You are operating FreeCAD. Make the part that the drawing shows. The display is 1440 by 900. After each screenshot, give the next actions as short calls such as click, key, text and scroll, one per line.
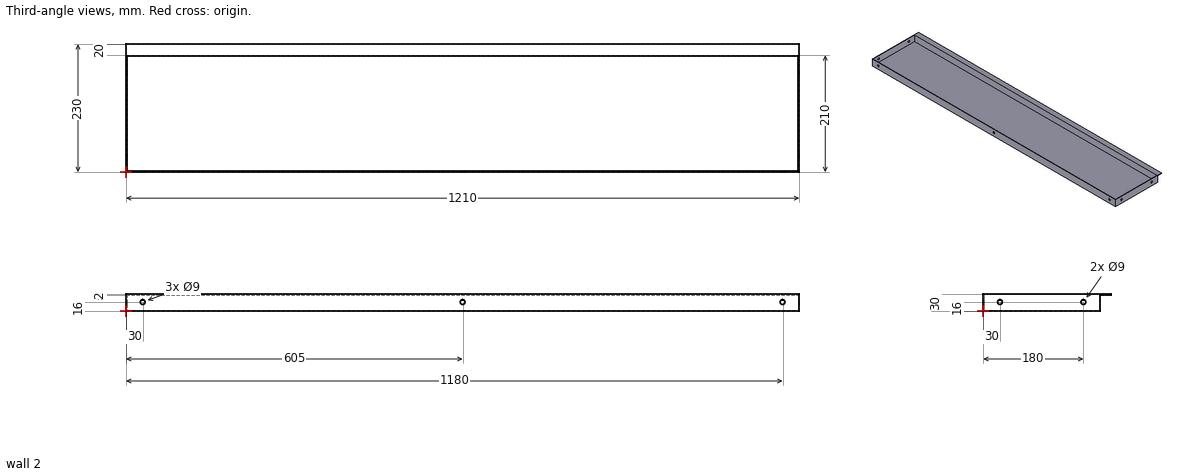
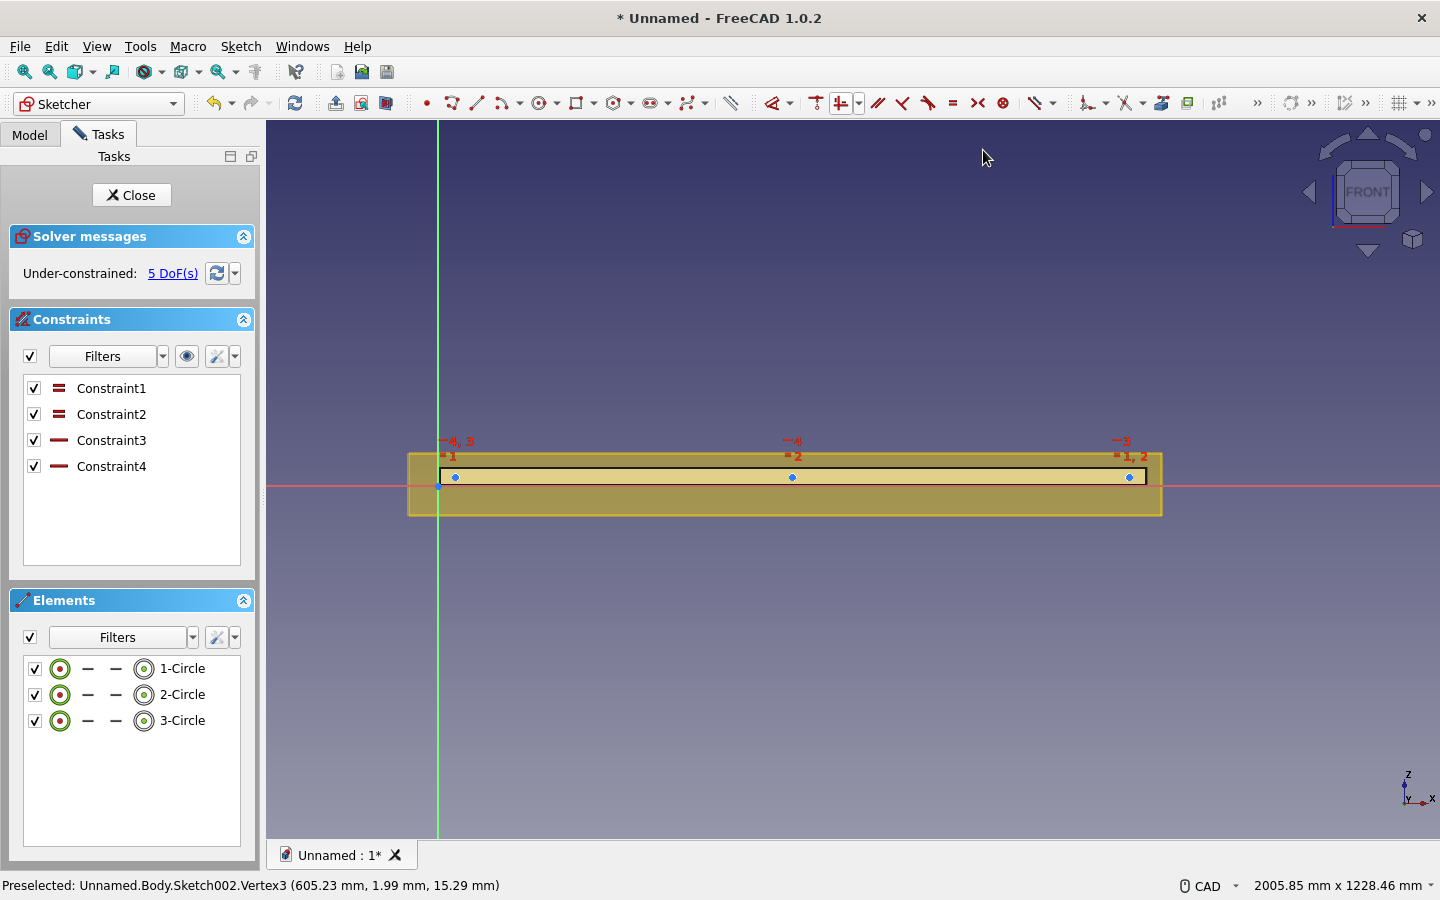
click(772, 104)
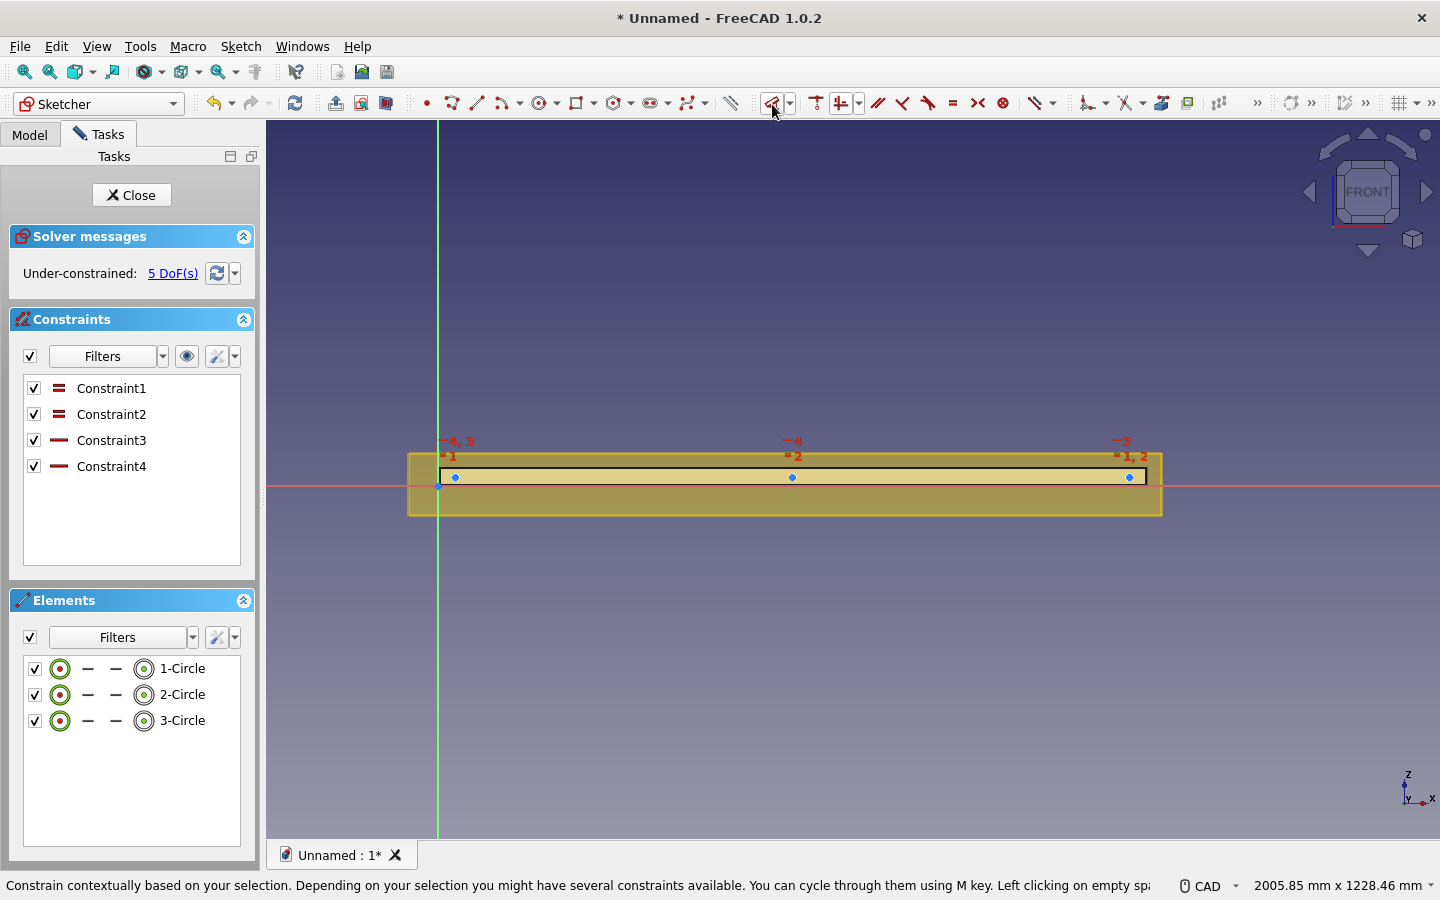
scroll(454, 475, up, 11)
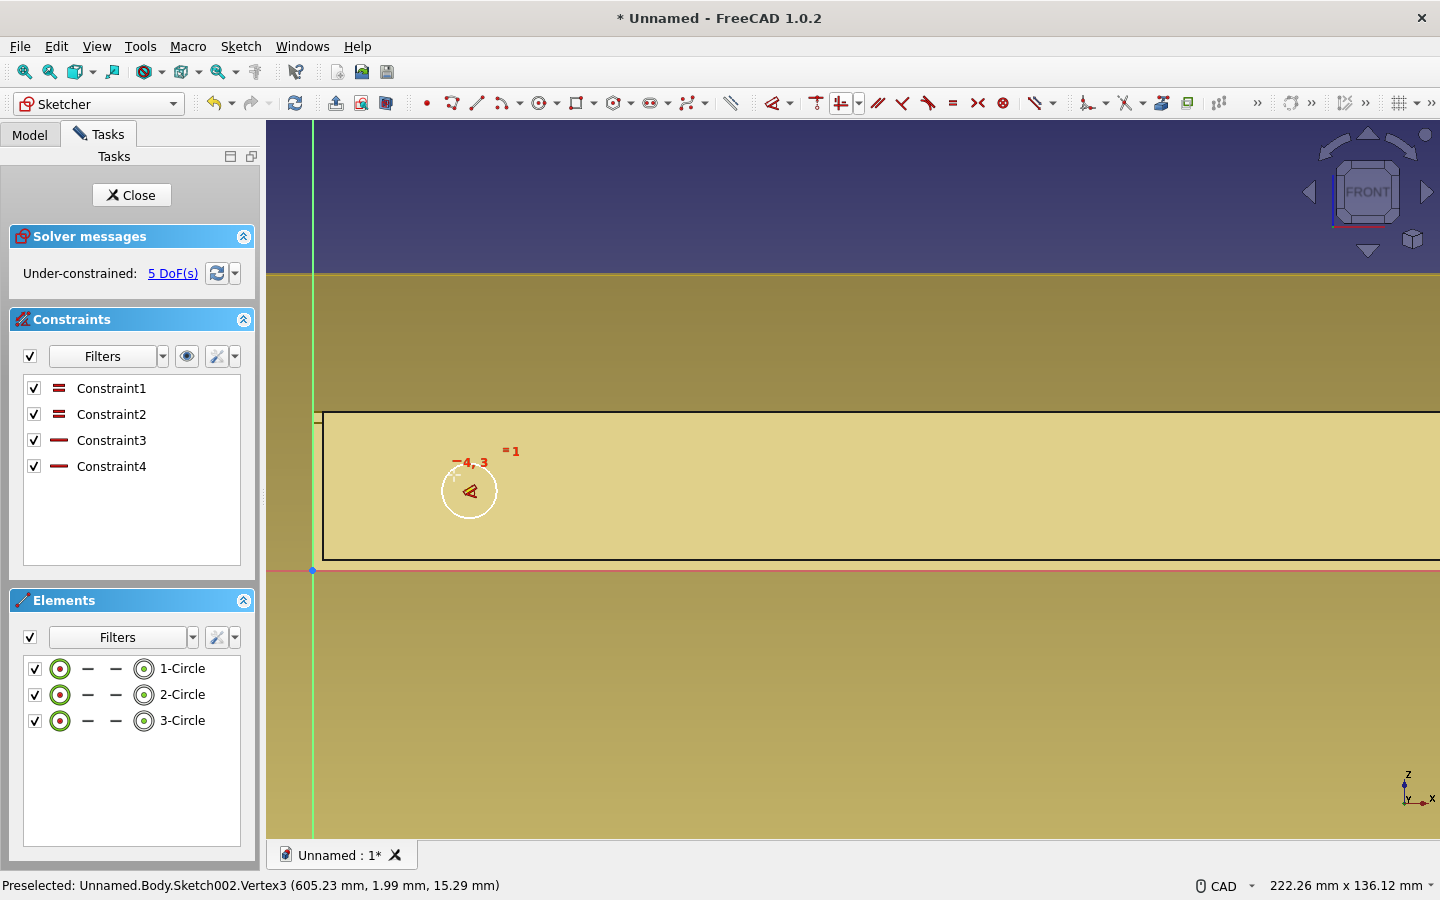
click(450, 472)
click(427, 450)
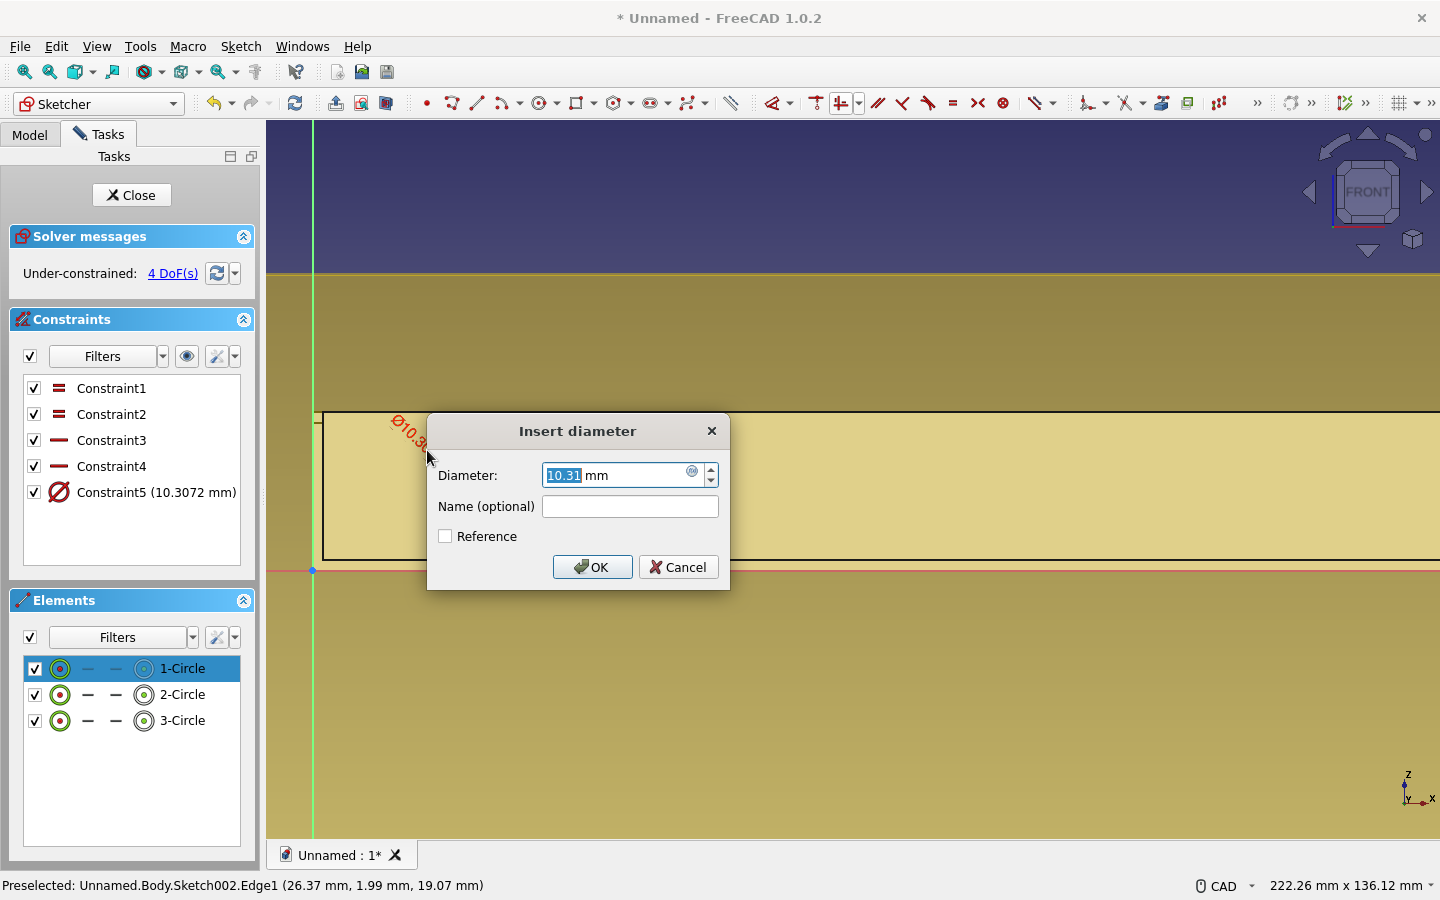
text(9)
key(Return)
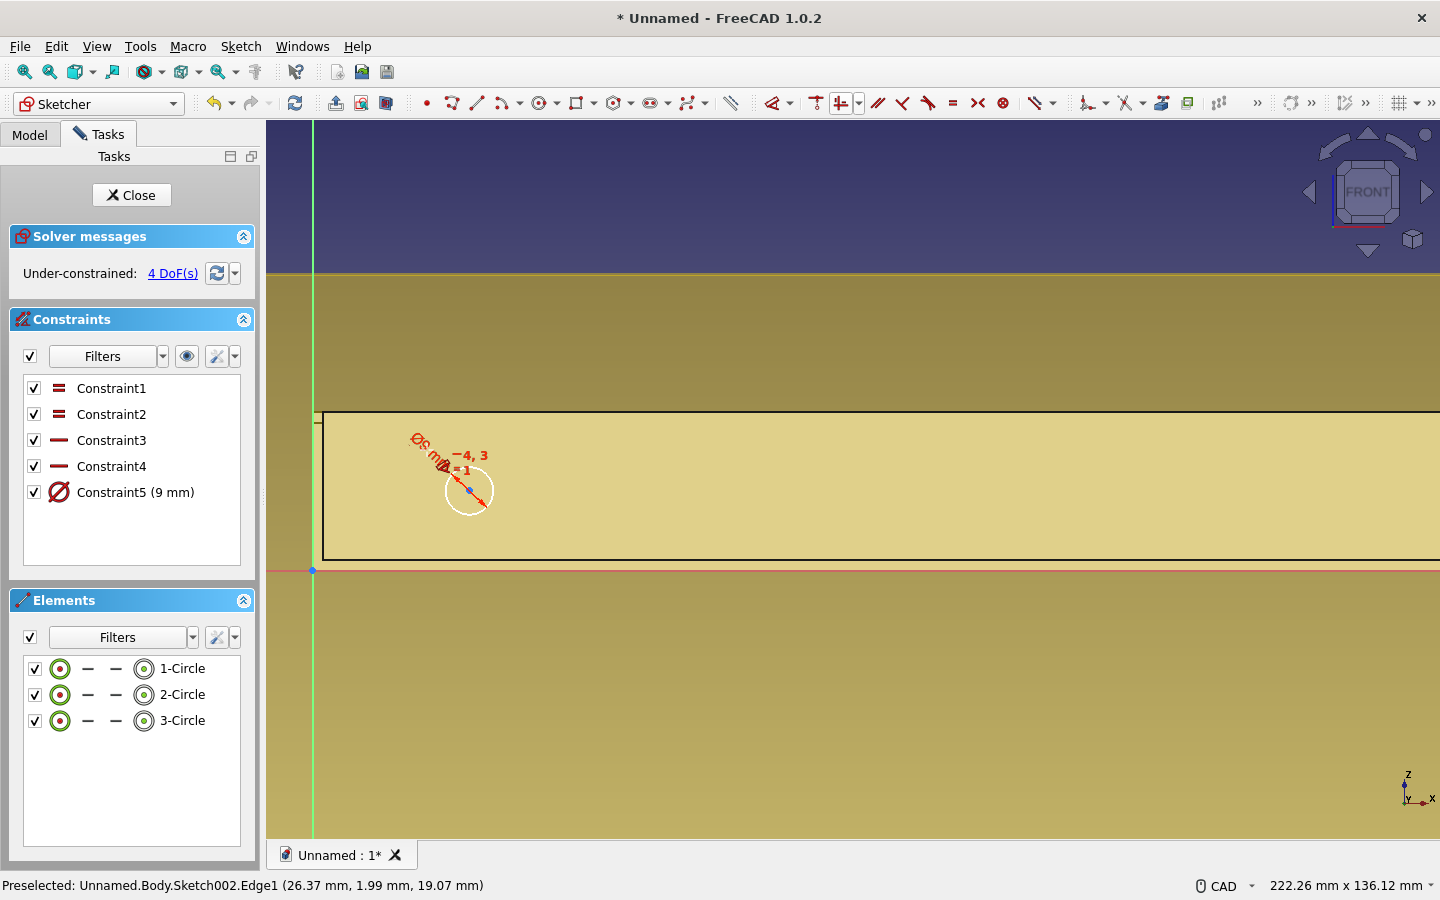
scroll(453, 475, down, 11)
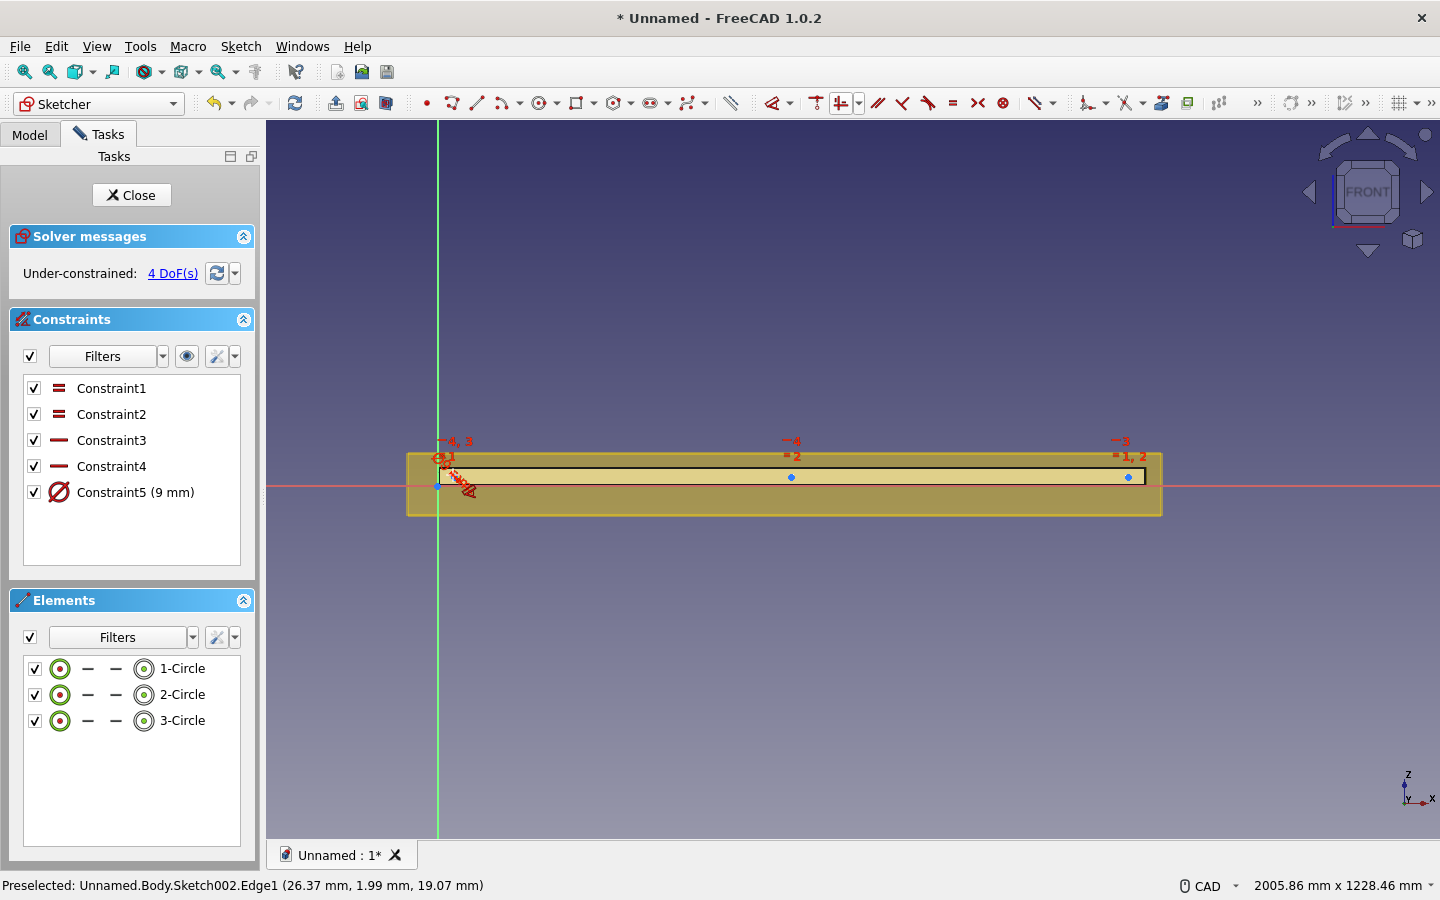
scroll(455, 477, up, 5)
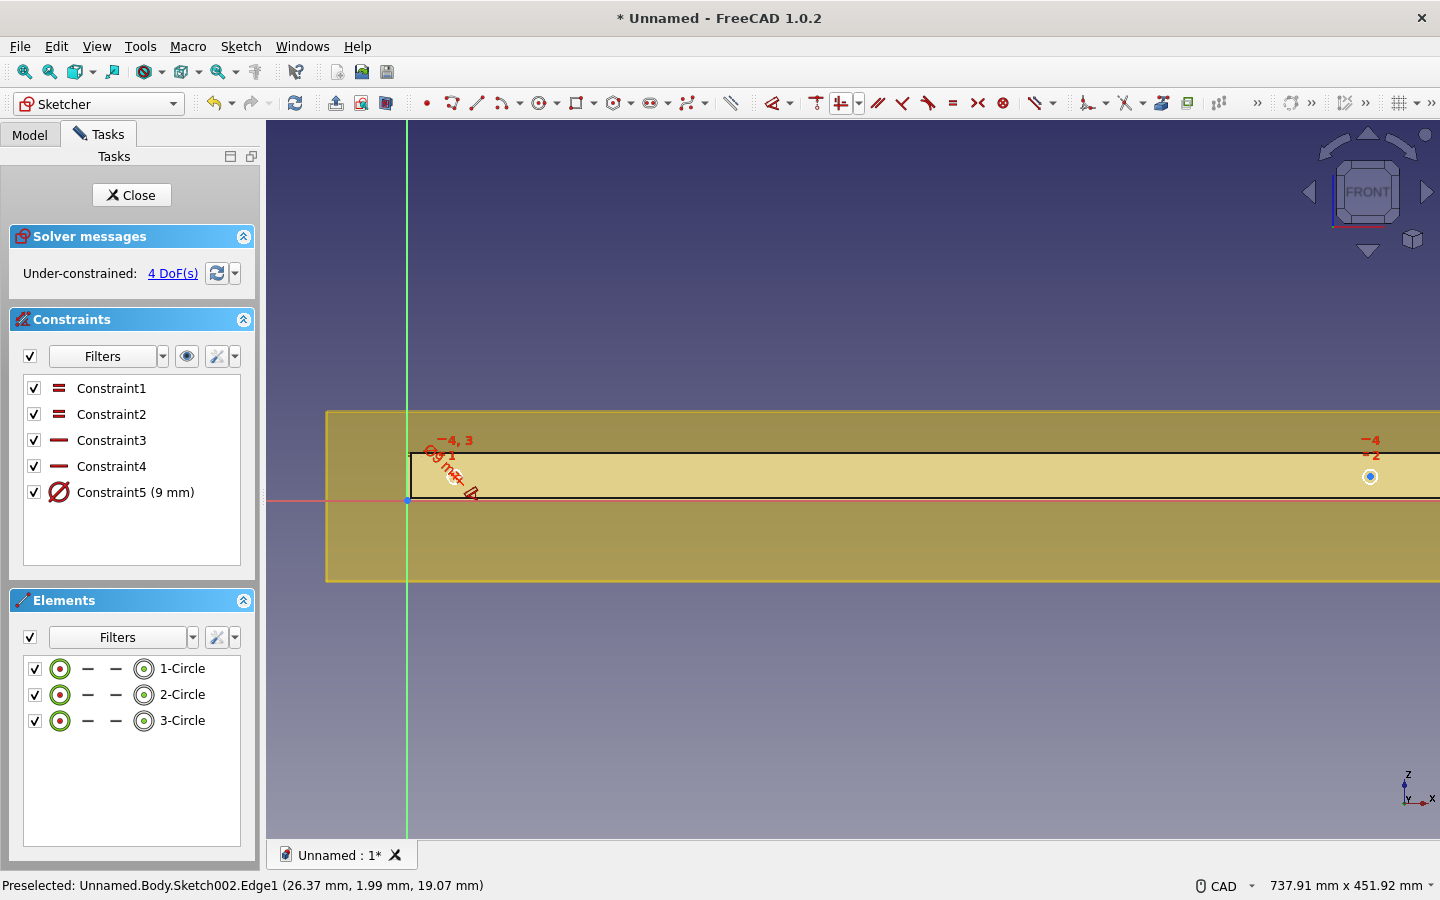
click(455, 477)
click(431, 535)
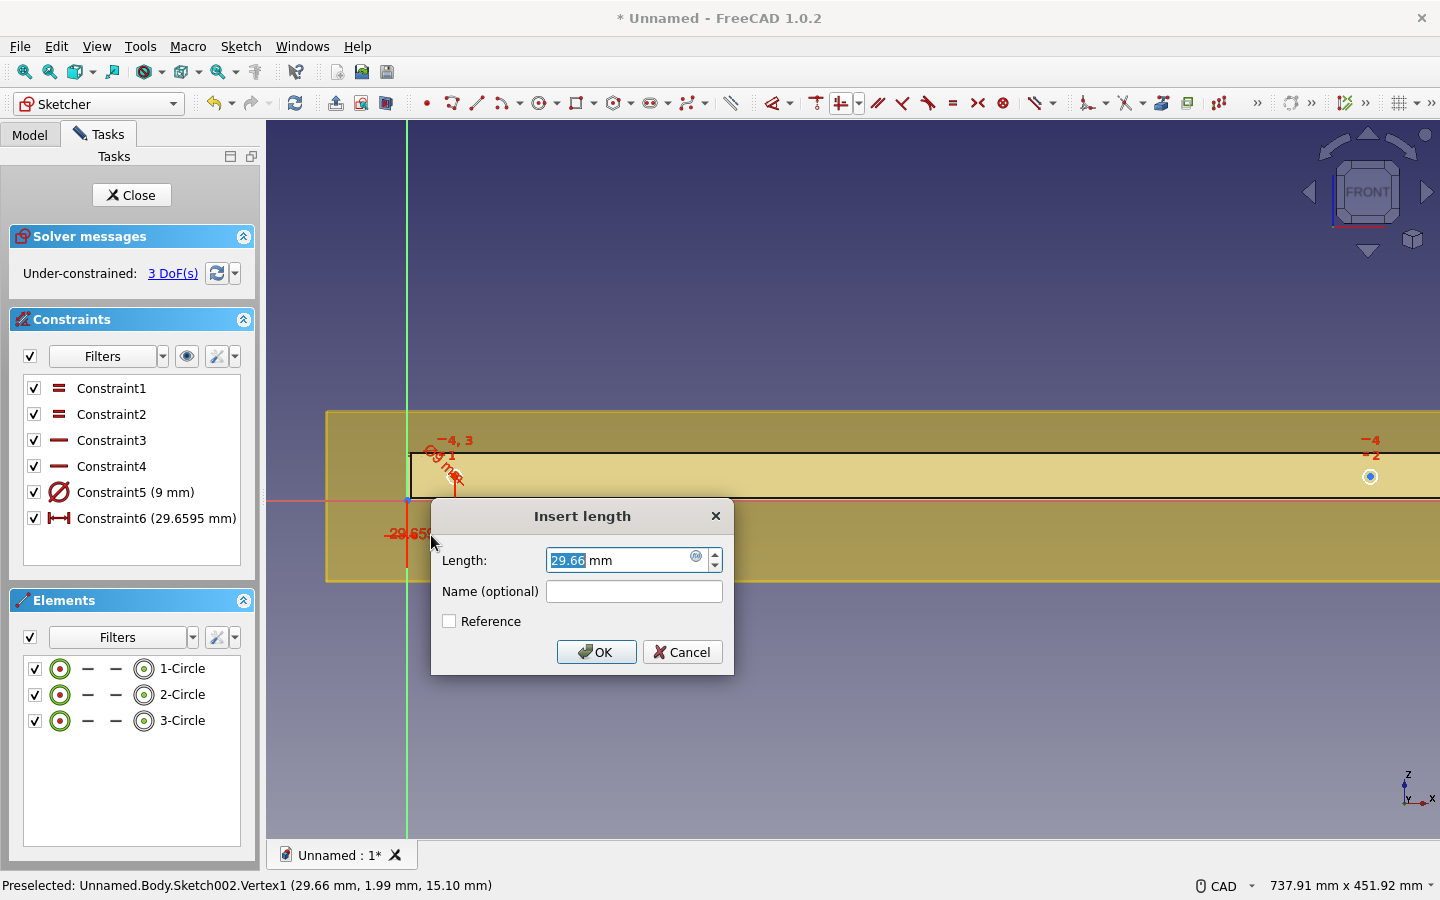
text(30)
key(Return)